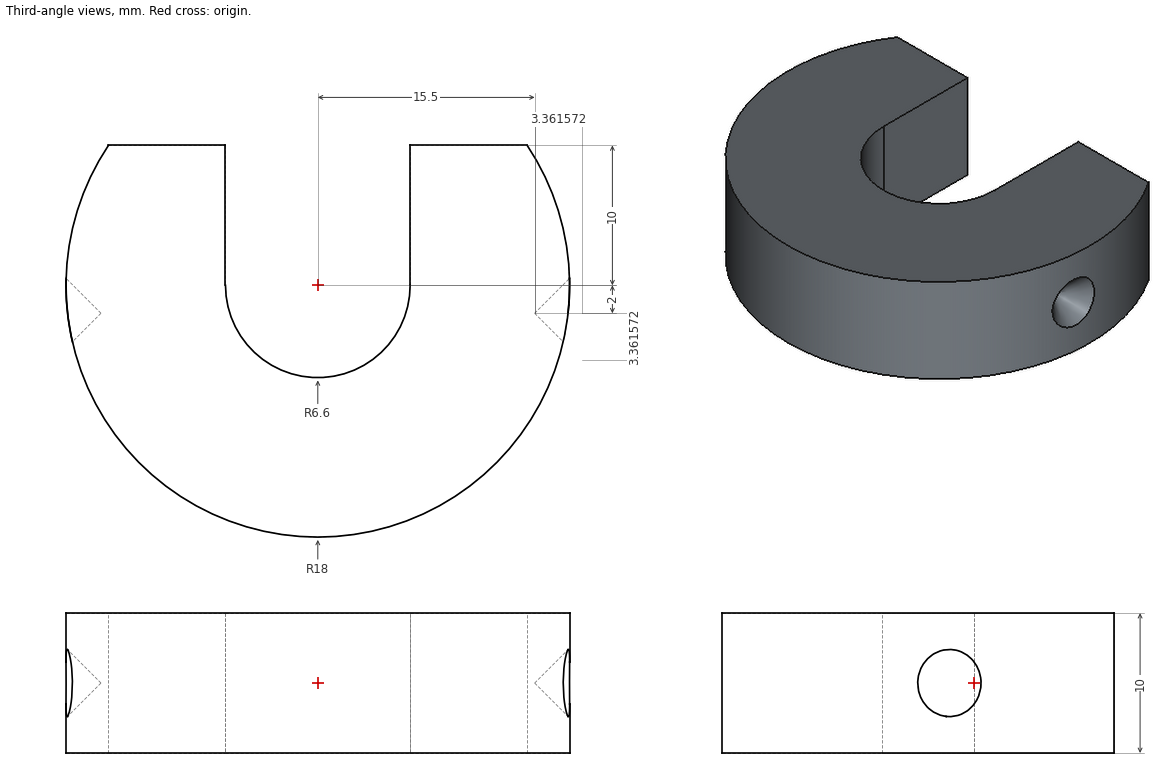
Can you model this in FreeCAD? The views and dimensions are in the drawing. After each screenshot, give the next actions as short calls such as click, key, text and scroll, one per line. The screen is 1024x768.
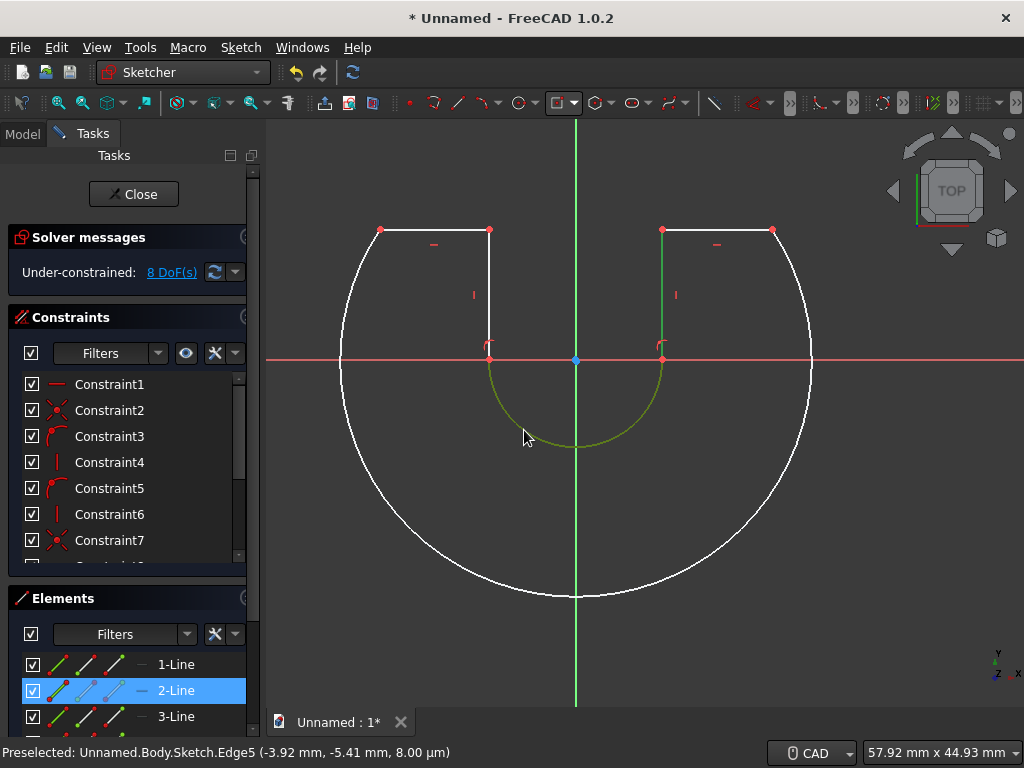
key(t)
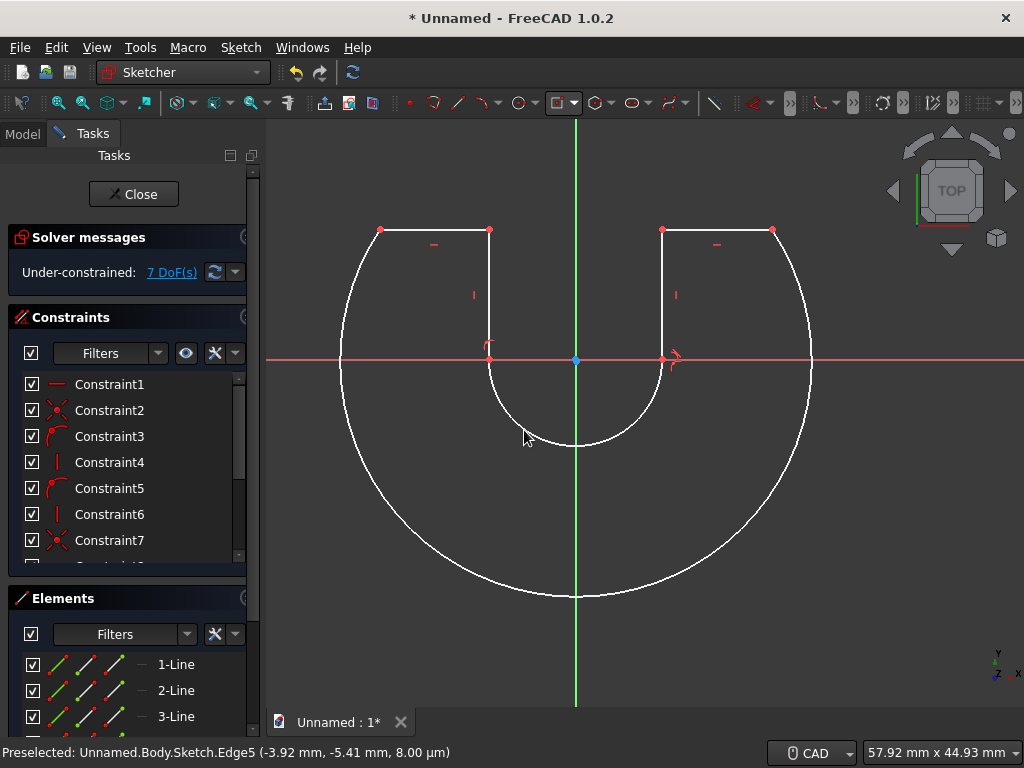
click(525, 430)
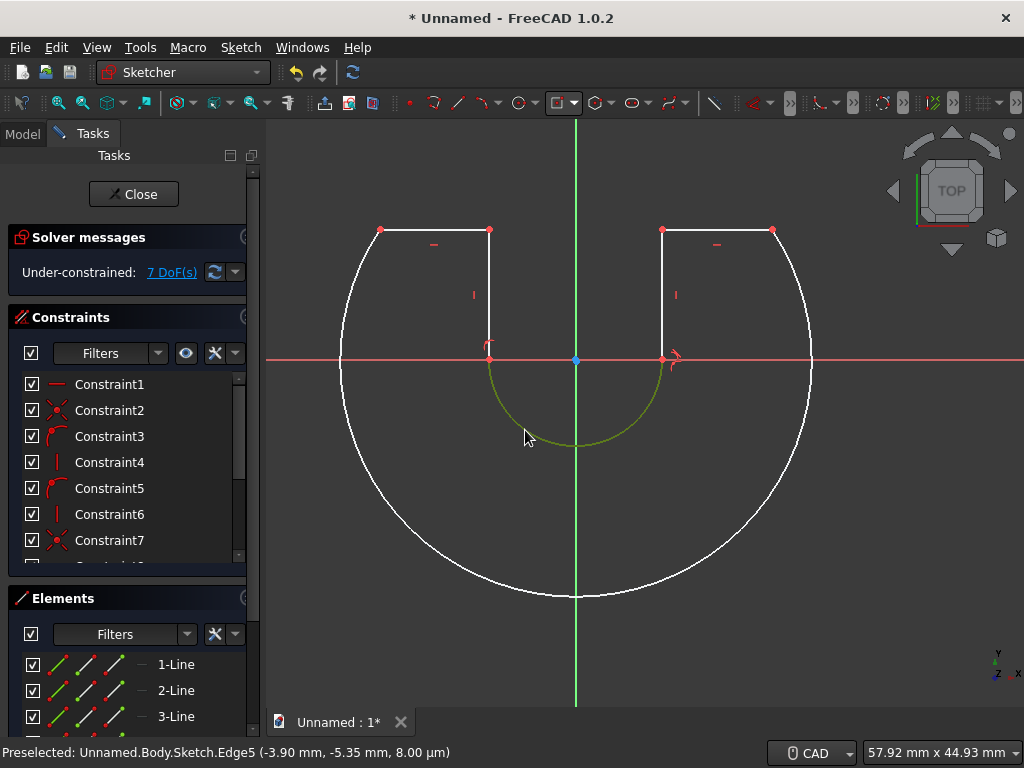
click(397, 514)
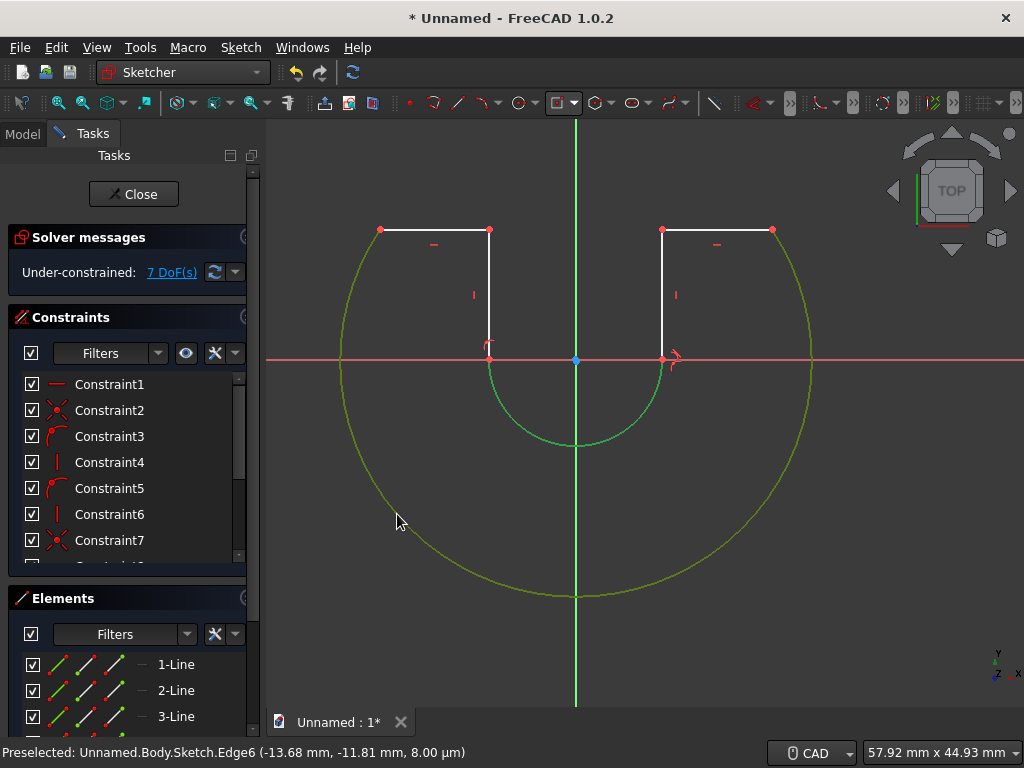
key(c)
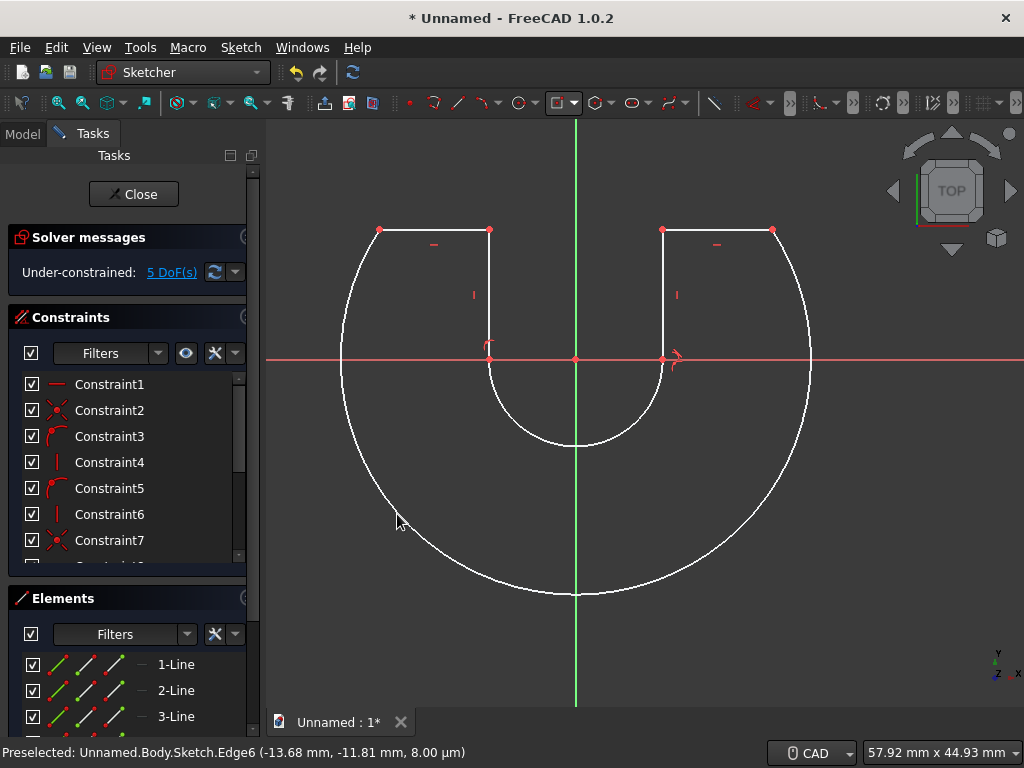
click(576, 360)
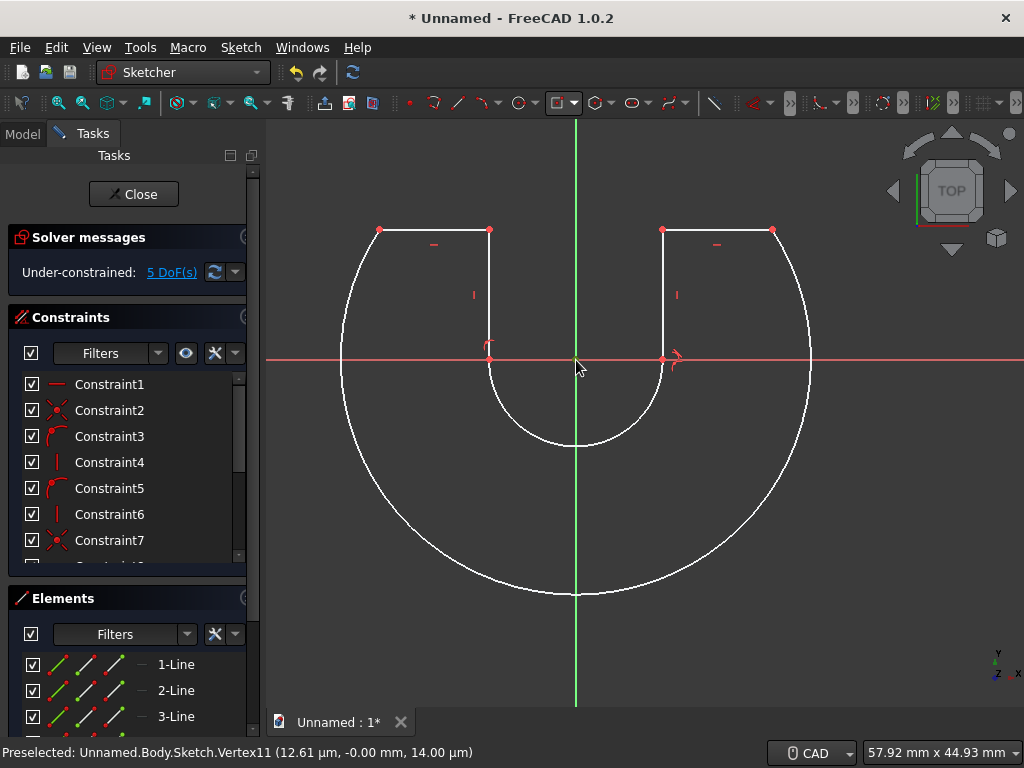
click(576, 641)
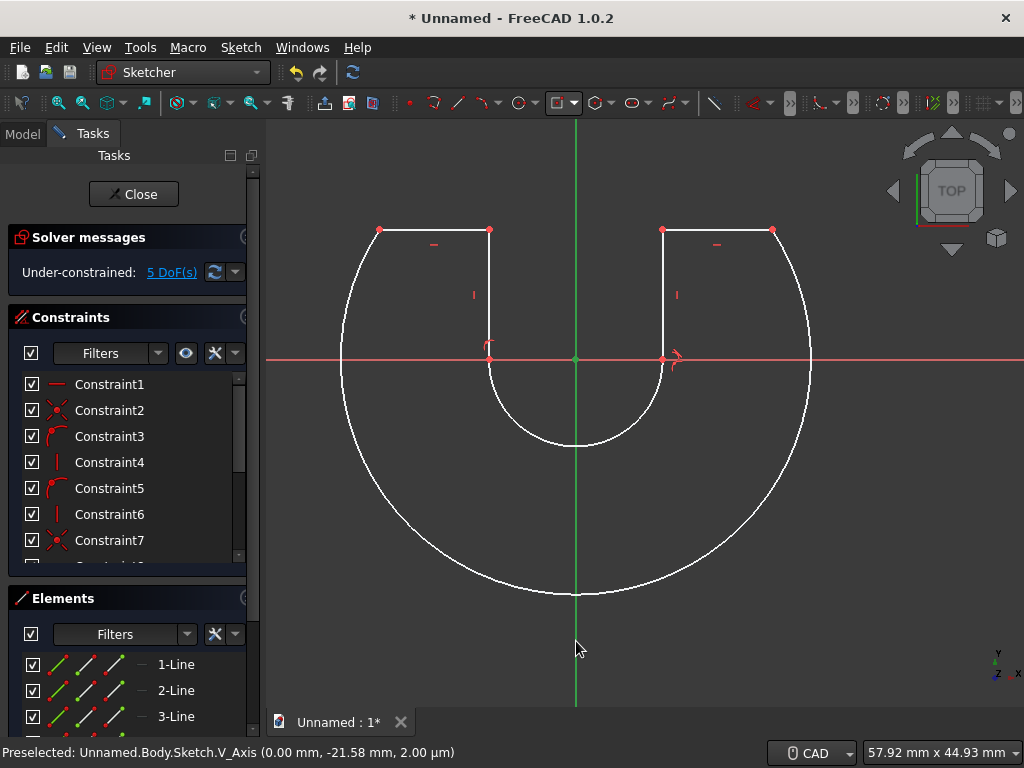
key(c)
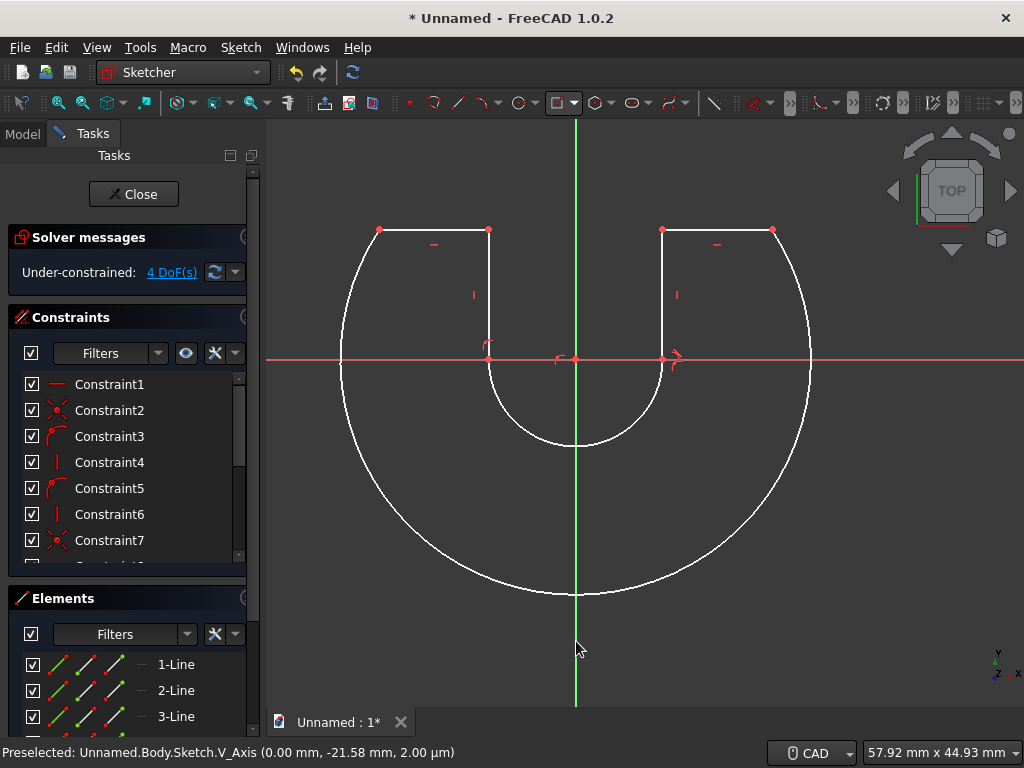
key(d)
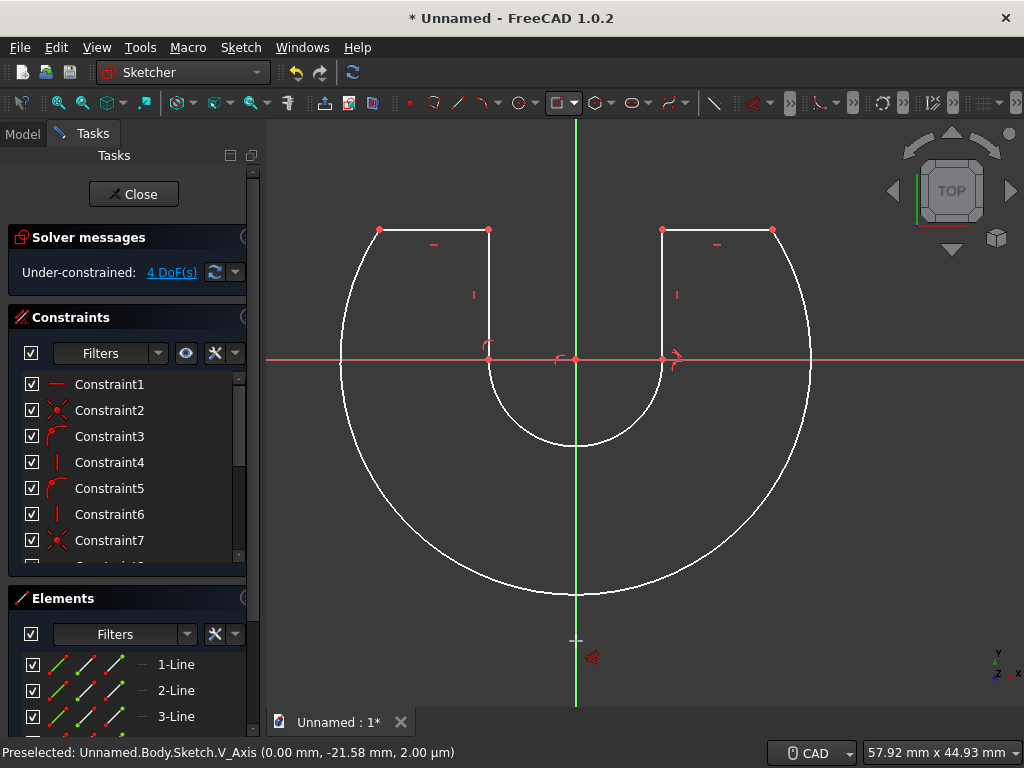
click(525, 430)
click(506, 456)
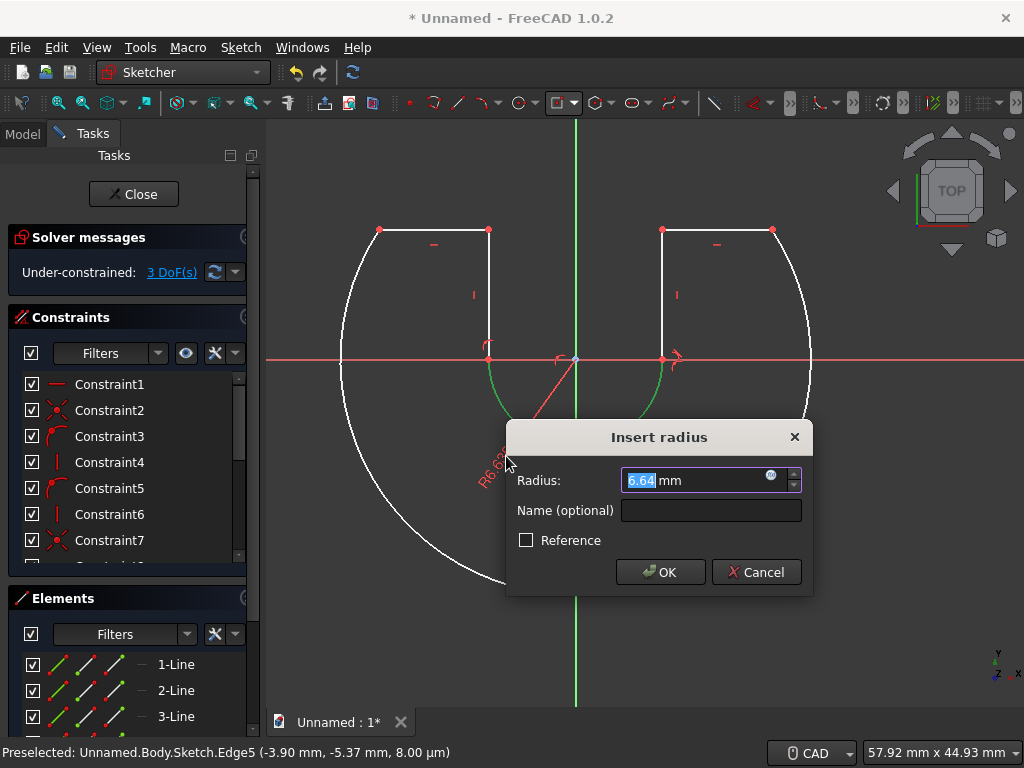
text(6.6)
key(Return)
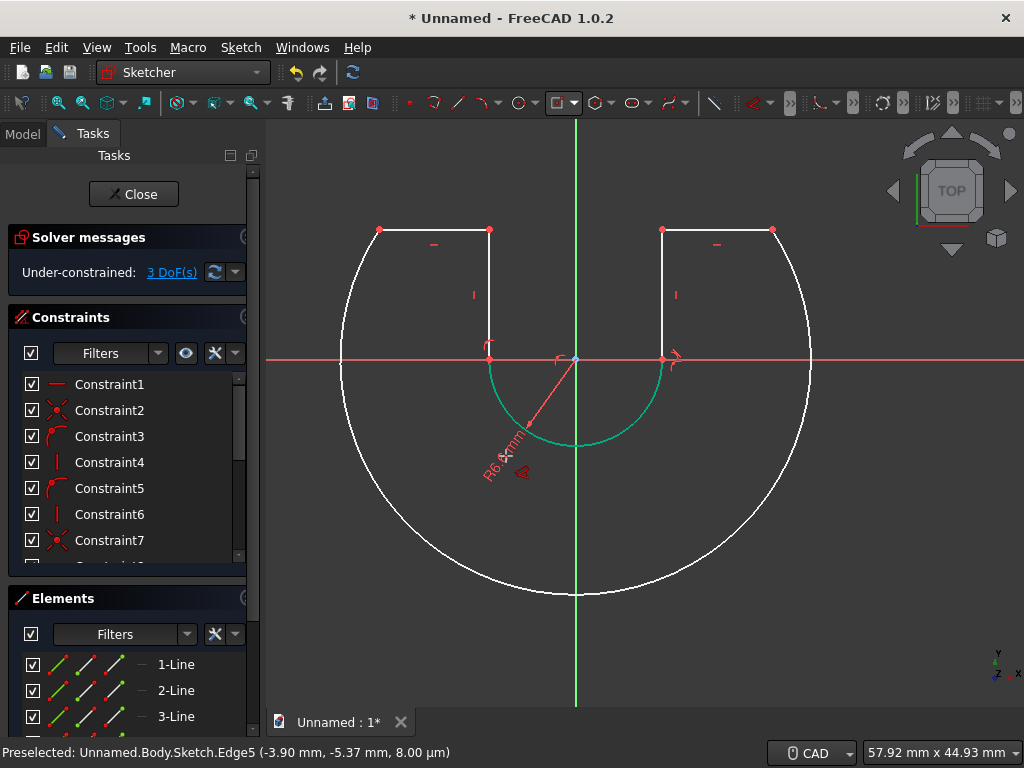
click(397, 513)
click(373, 534)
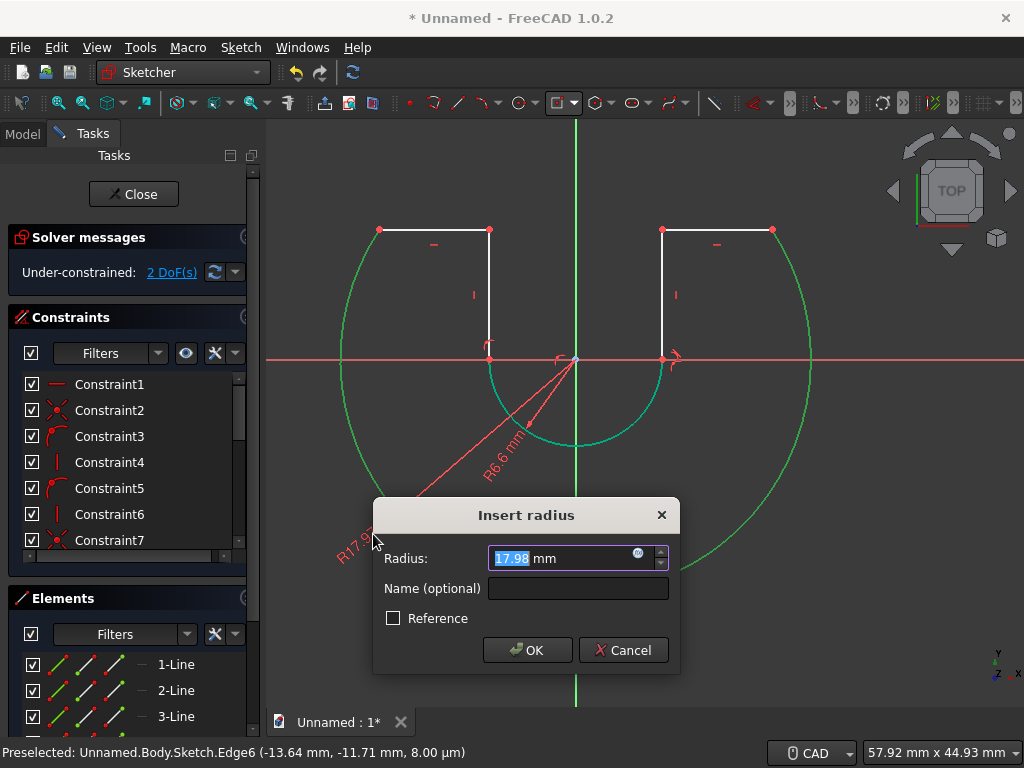
text(18)
key(Return)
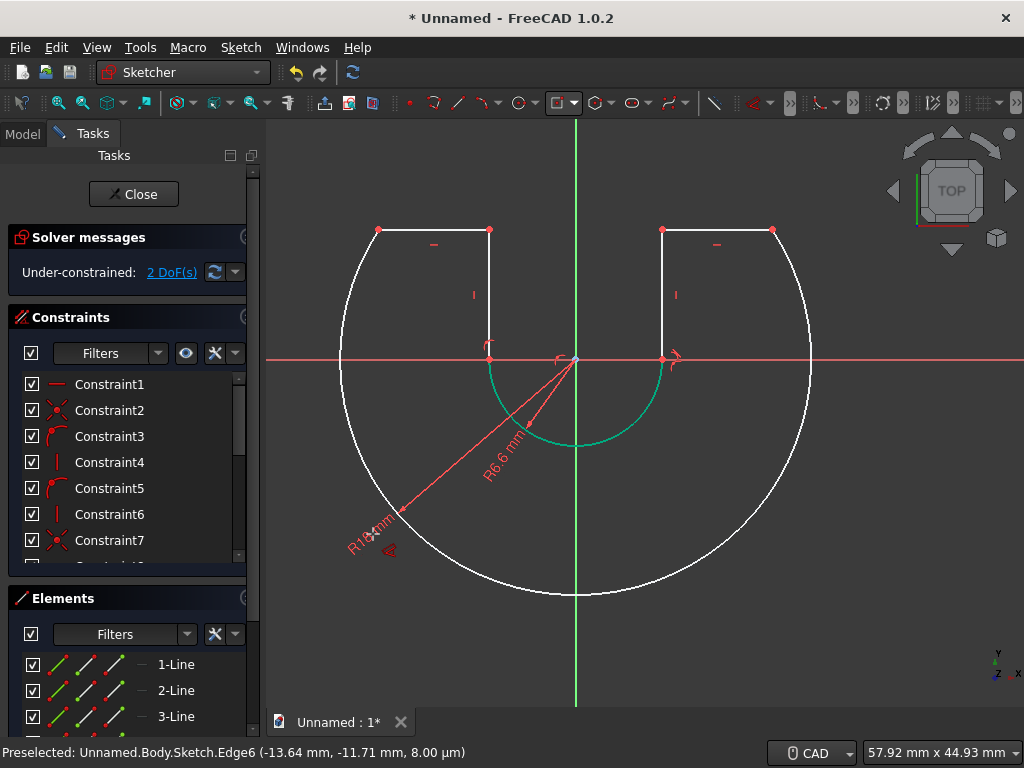
click(662, 269)
click(696, 295)